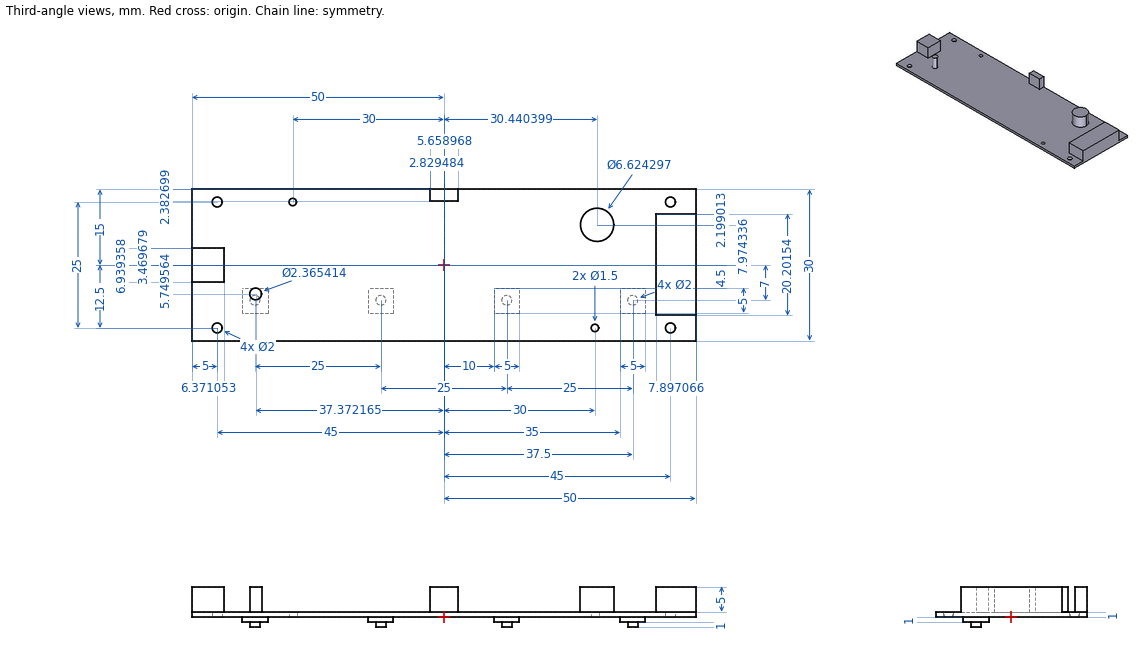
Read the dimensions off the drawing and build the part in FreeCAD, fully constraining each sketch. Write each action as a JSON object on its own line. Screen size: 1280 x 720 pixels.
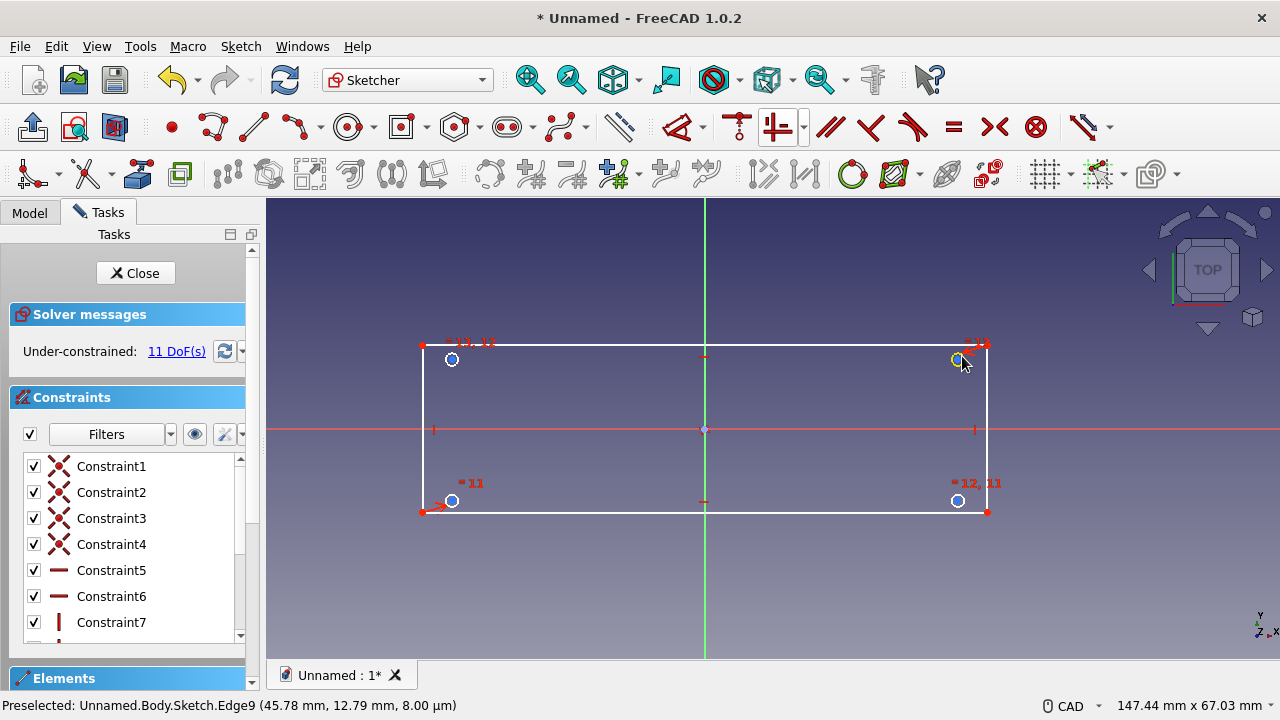
{"action": "left_click", "coordinate": [452, 501]}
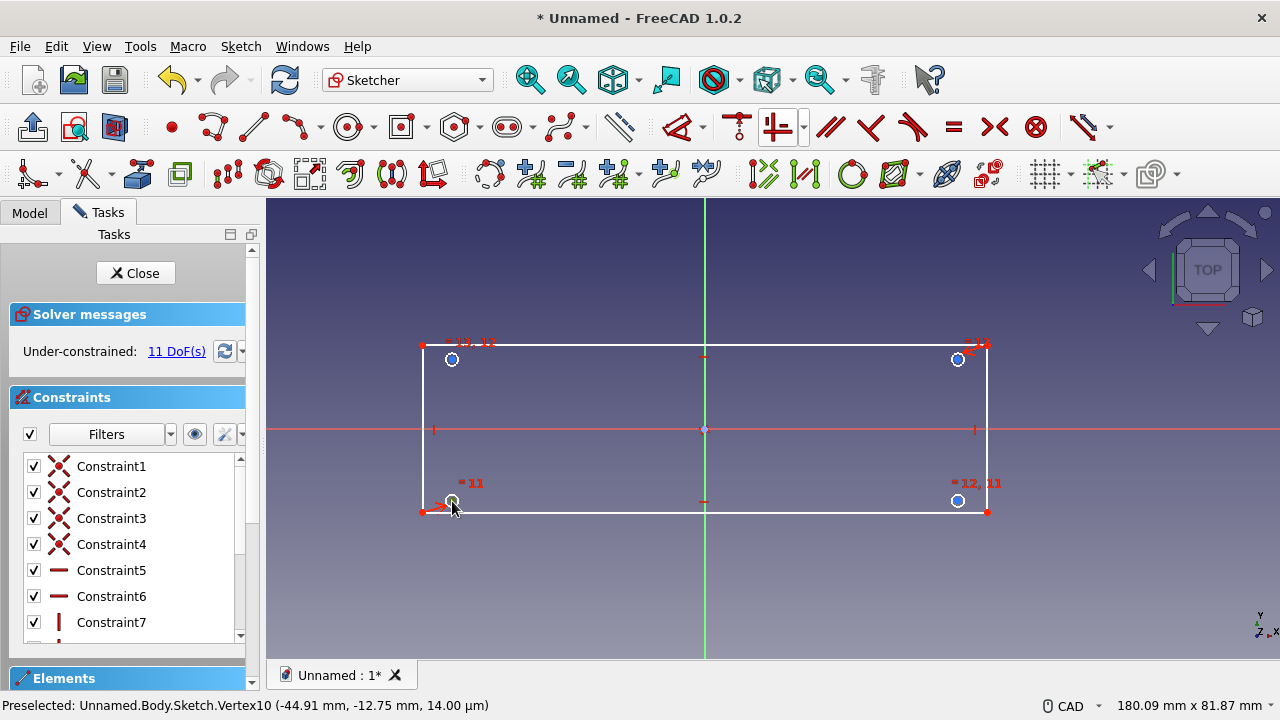
{"action": "left_click", "coordinate": [958, 501]}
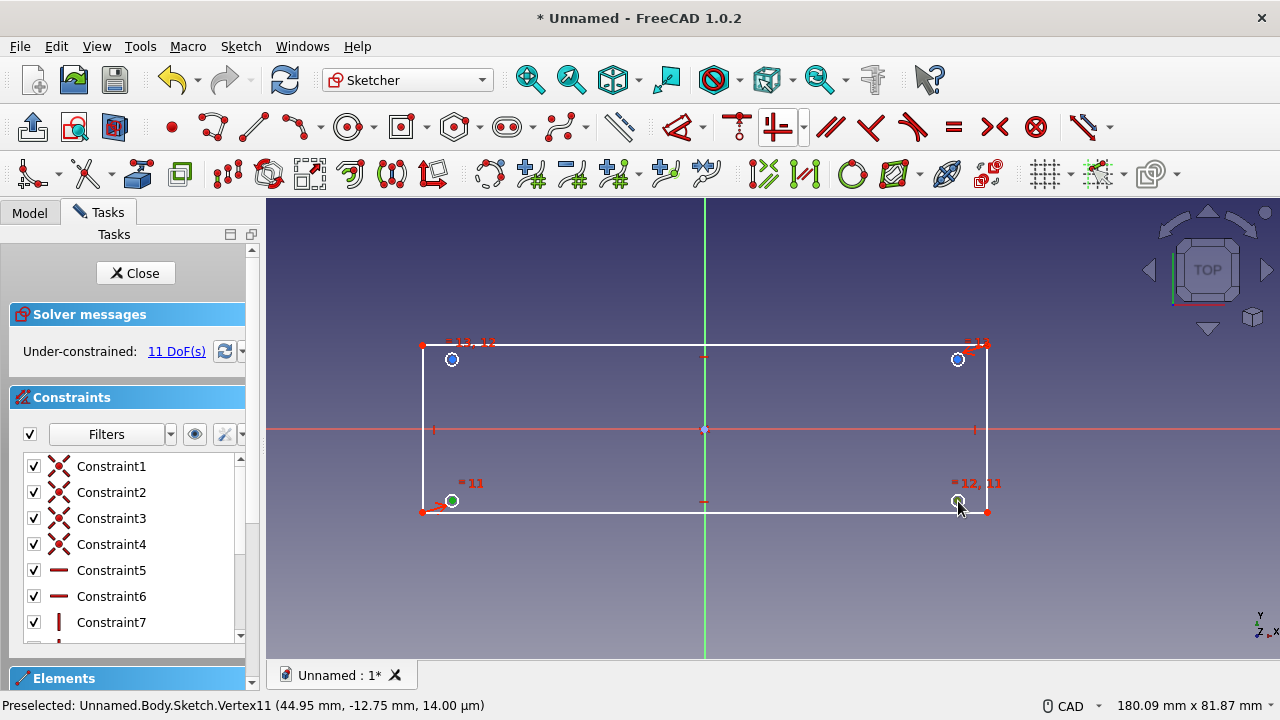
{"action": "key", "text": "h"}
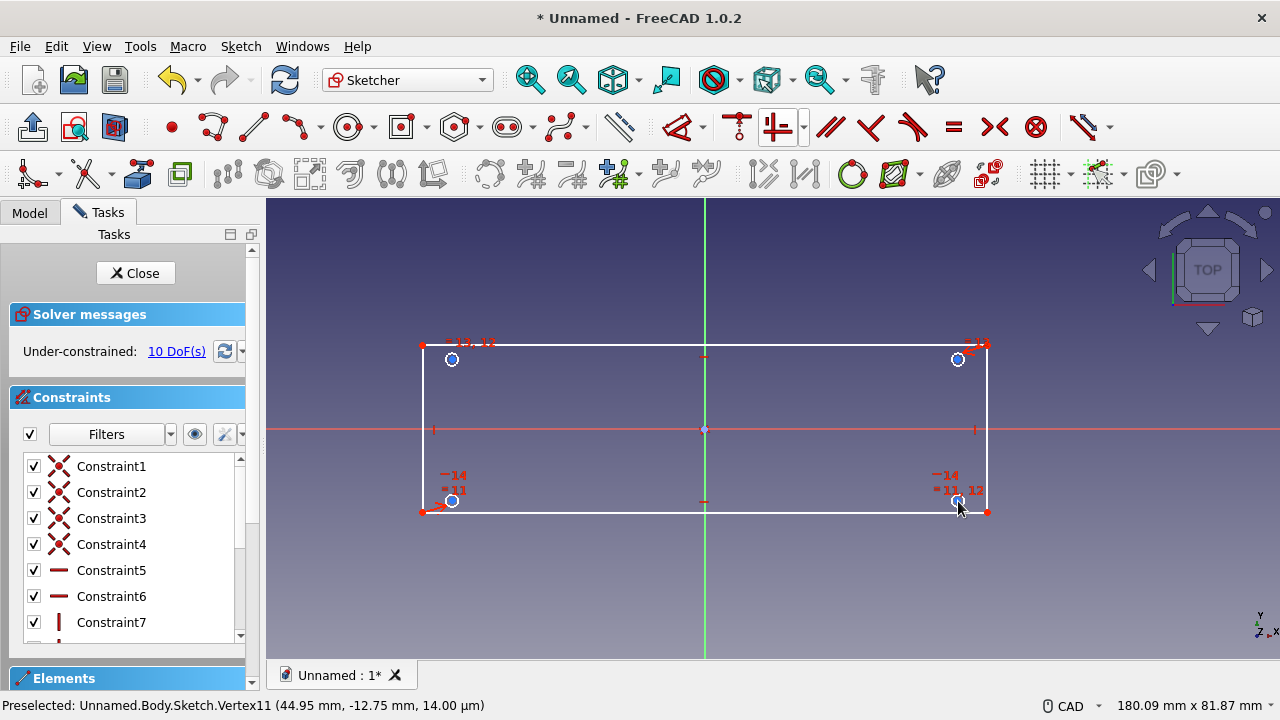
{"action": "left_click", "coordinate": [452, 501]}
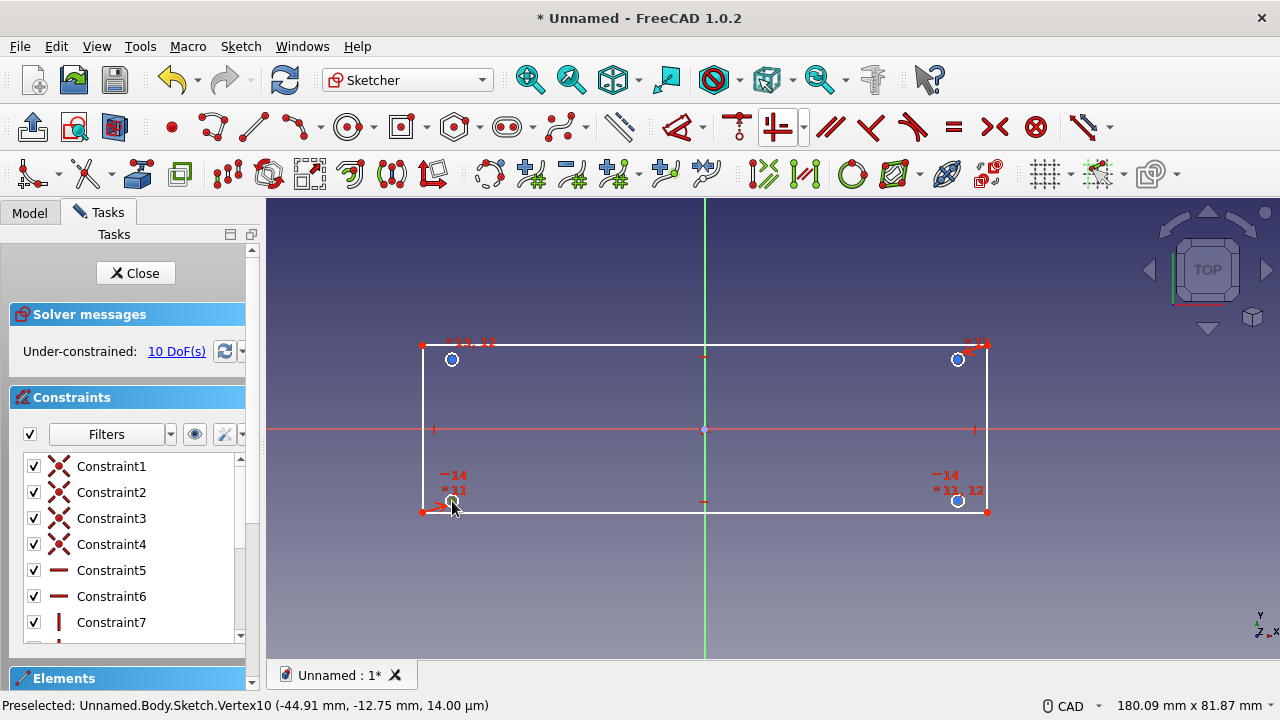
{"action": "left_click", "coordinate": [452, 360]}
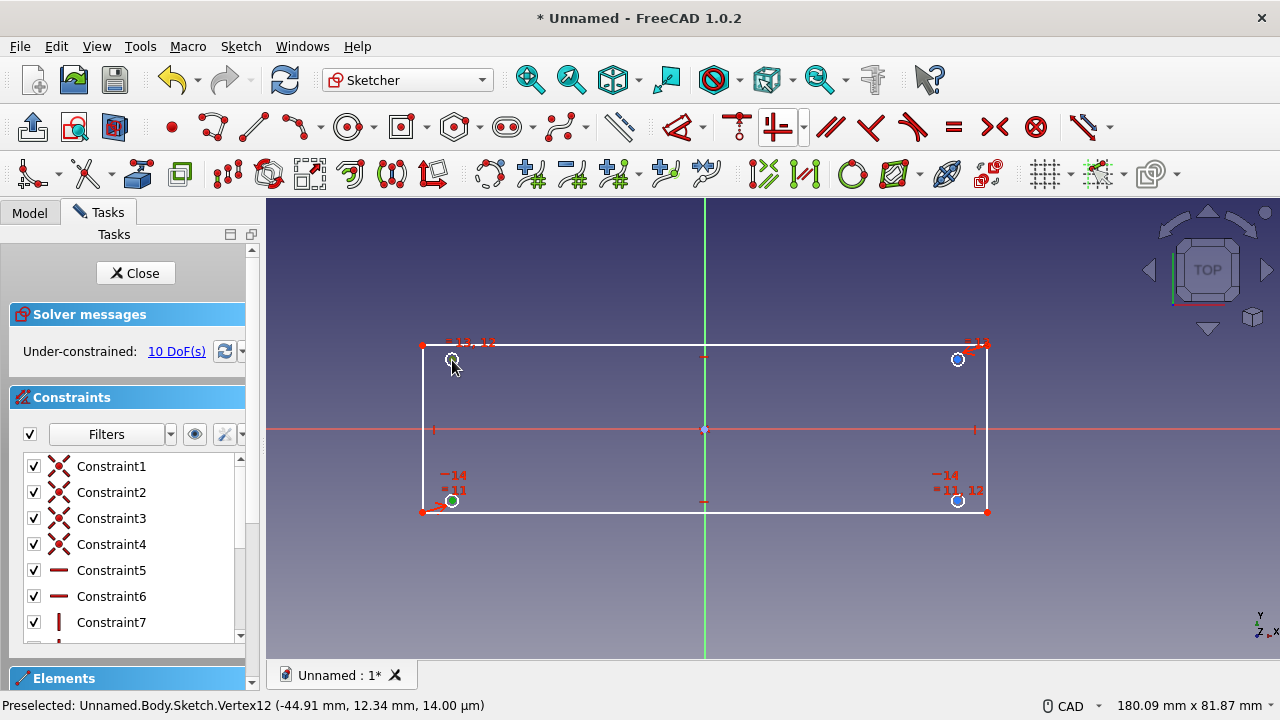
{"action": "left_click", "coordinate": [804, 128]}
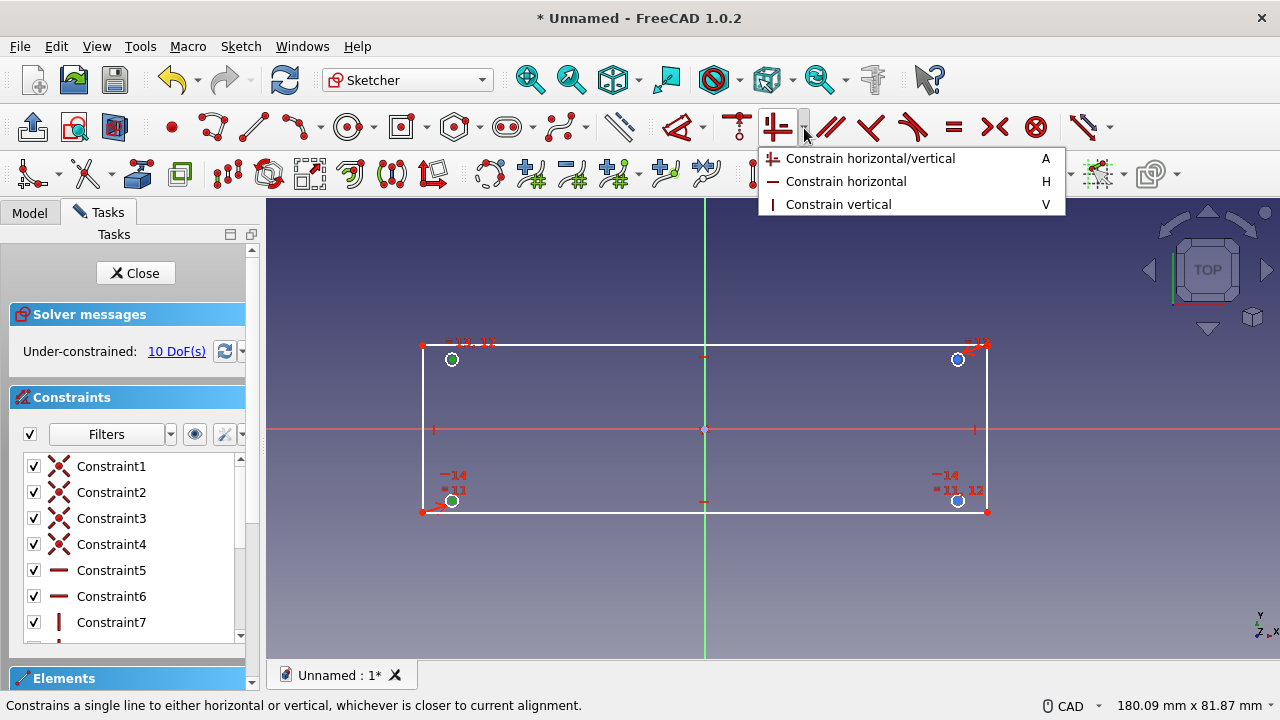
{"action": "left_click", "coordinate": [912, 204]}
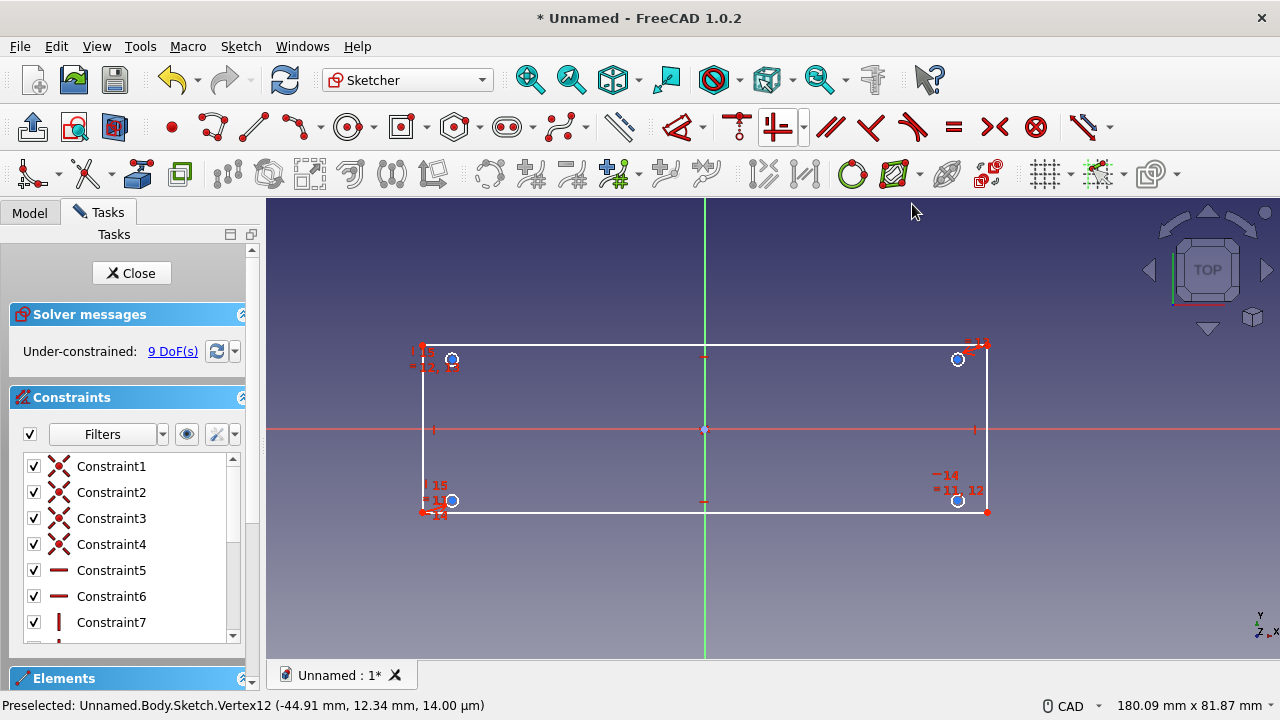
{"action": "left_click", "coordinate": [958, 501]}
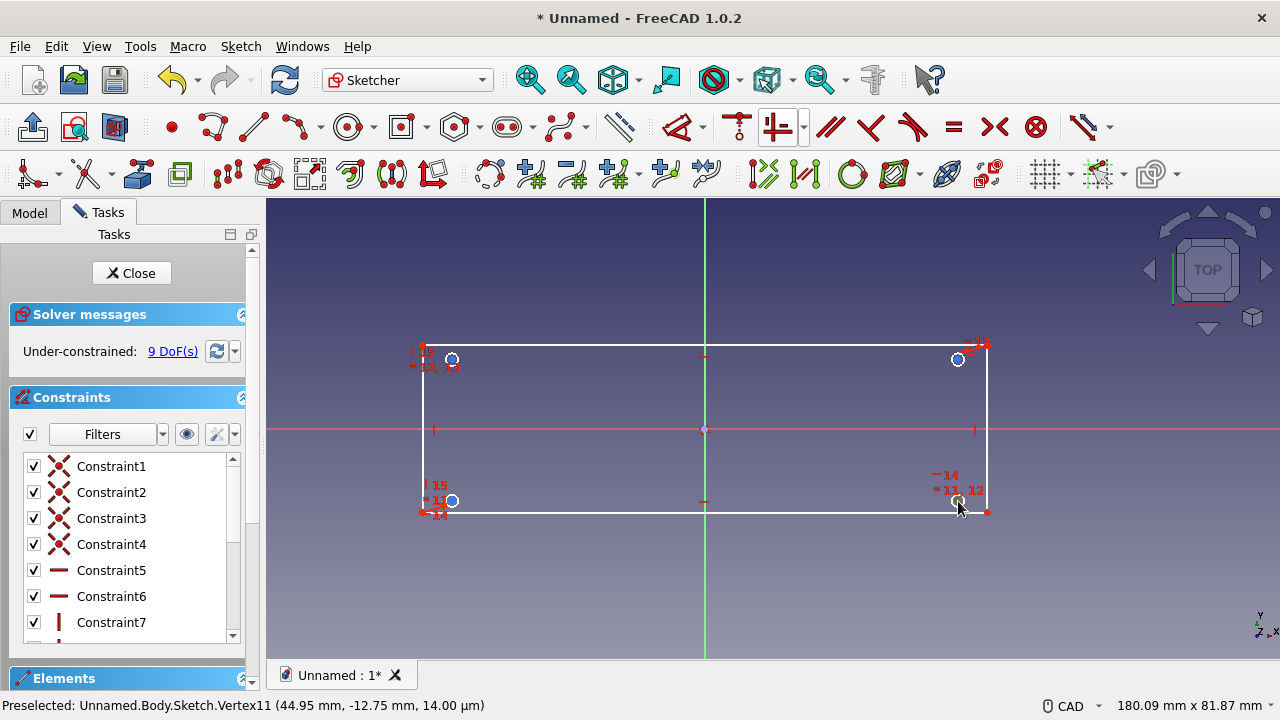
{"action": "left_click", "coordinate": [958, 360]}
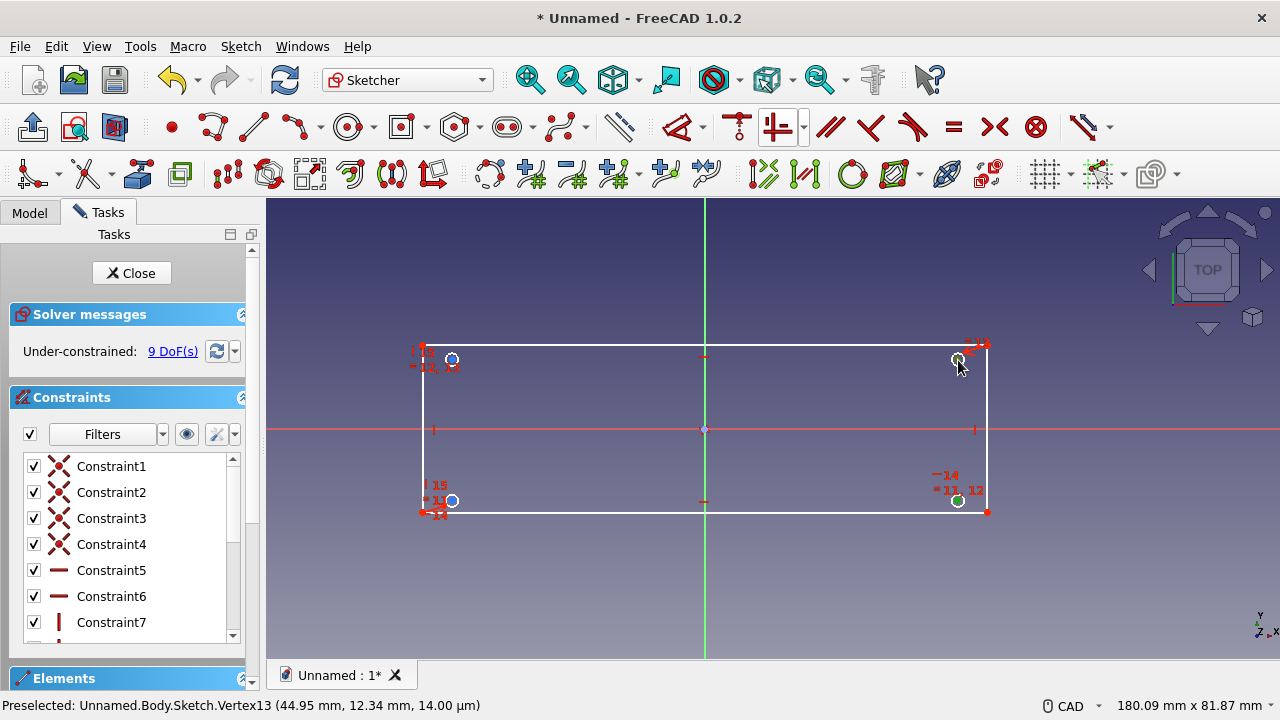
{"action": "left_click", "coordinate": [804, 128]}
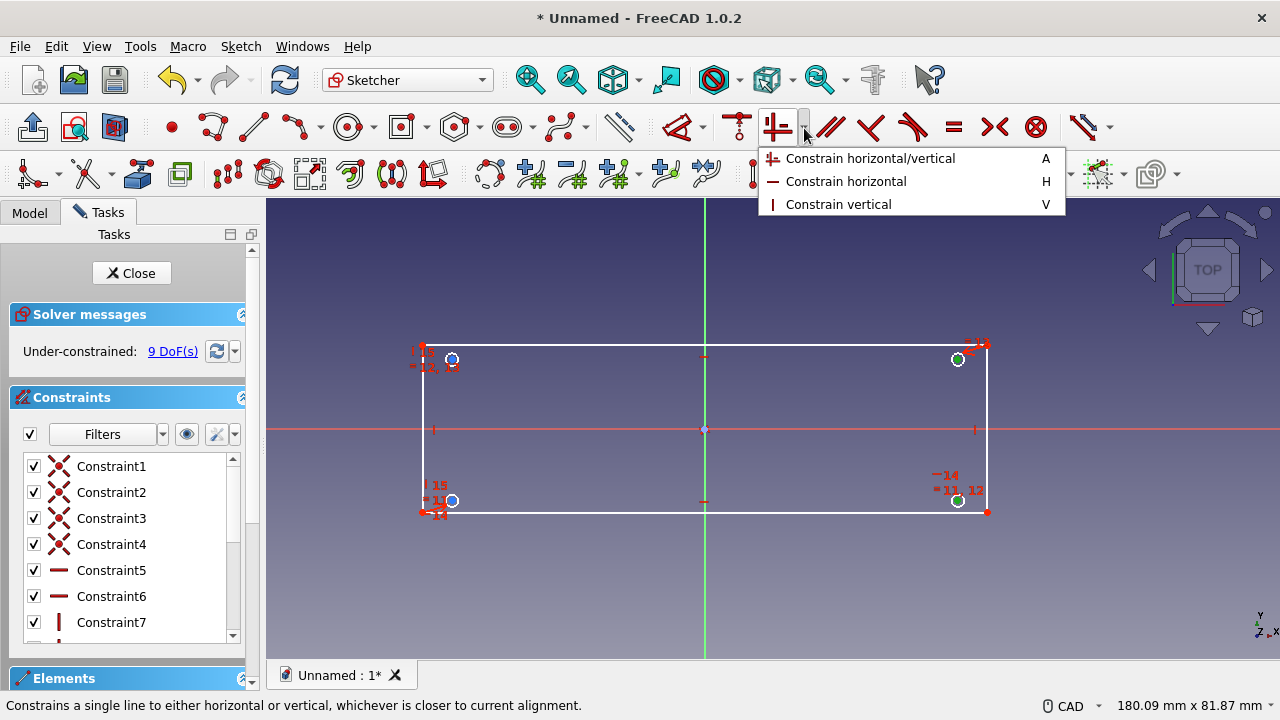
{"action": "left_click", "coordinate": [912, 204]}